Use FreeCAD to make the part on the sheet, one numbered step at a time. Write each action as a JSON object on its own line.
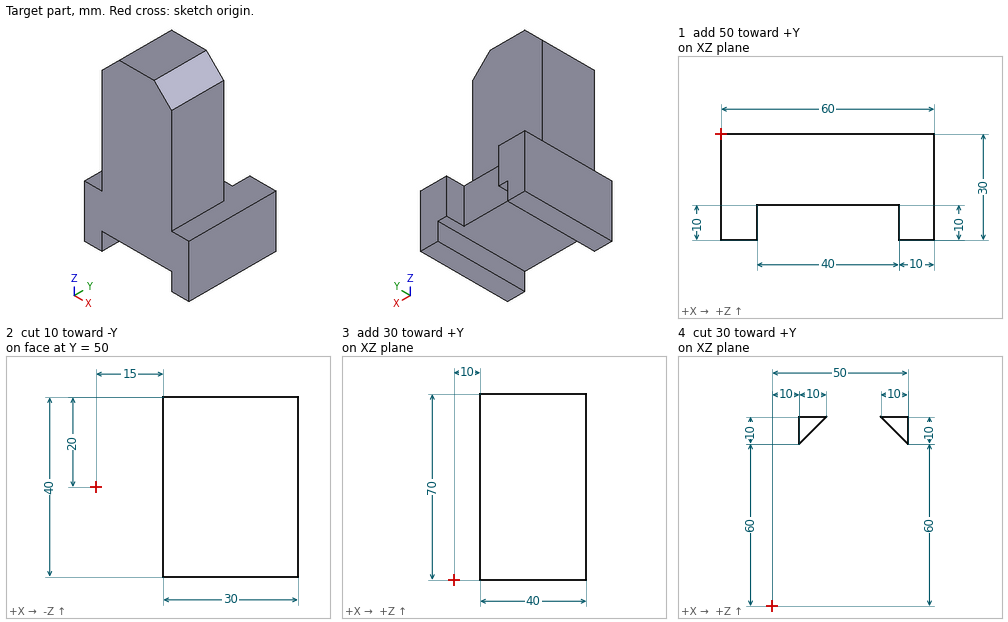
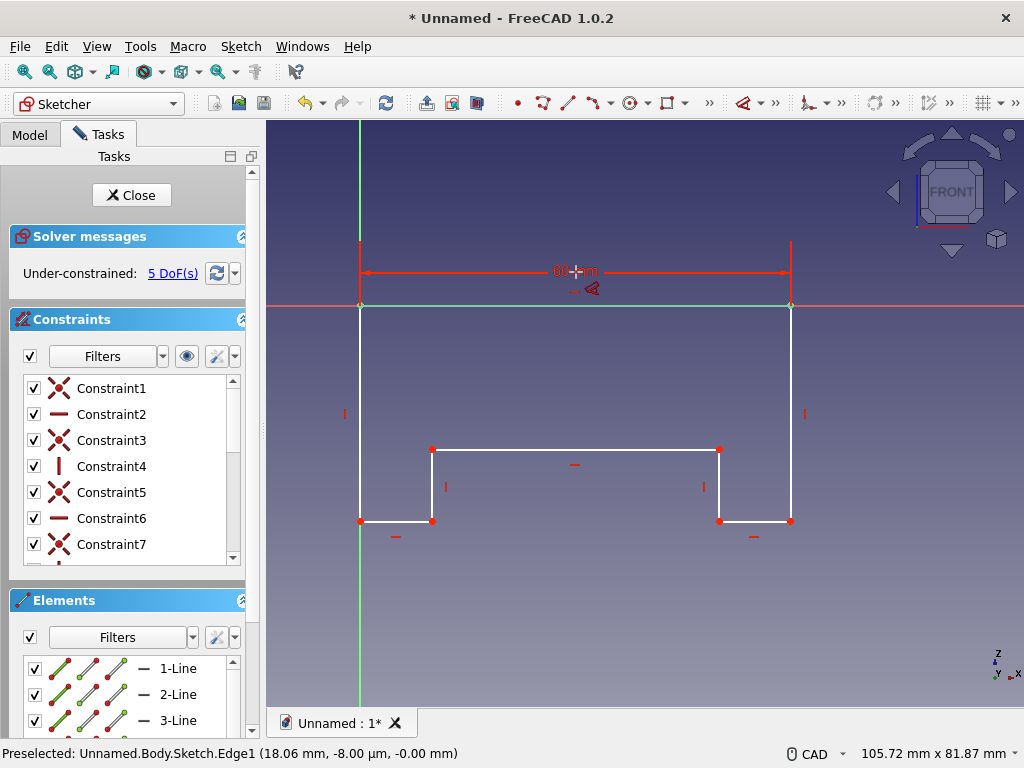
{"action": "left_click", "coordinate": [791, 371]}
{"action": "left_click", "coordinate": [825, 414]}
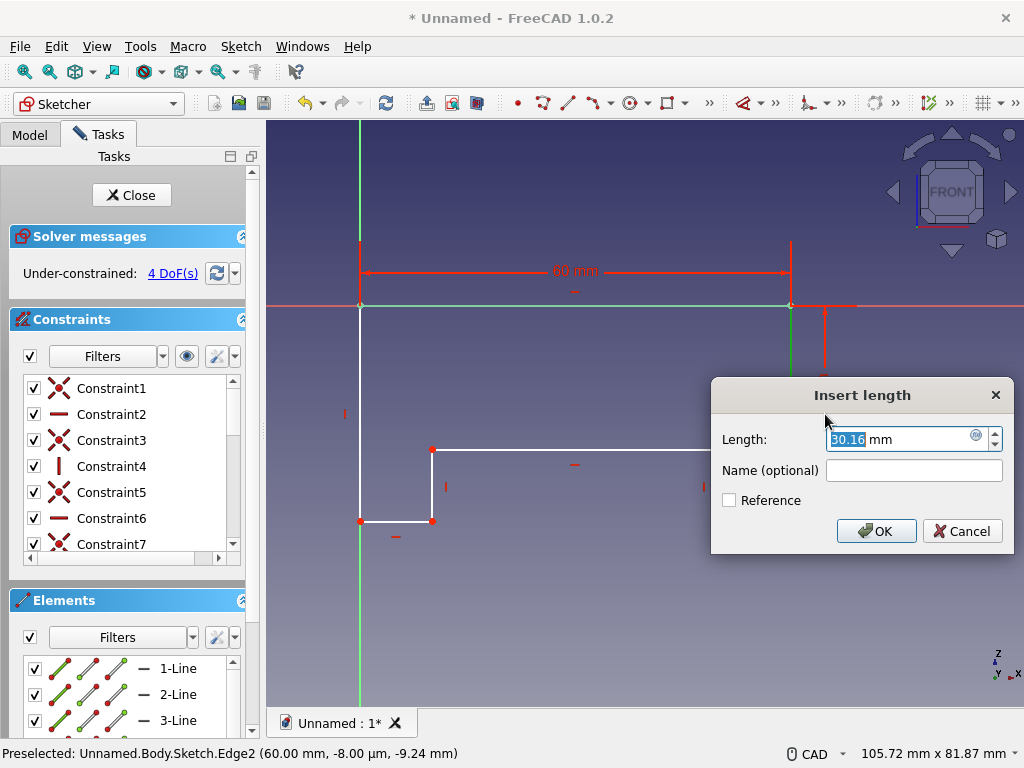
{"action": "type", "text": "30"}
{"action": "key", "text": "Return"}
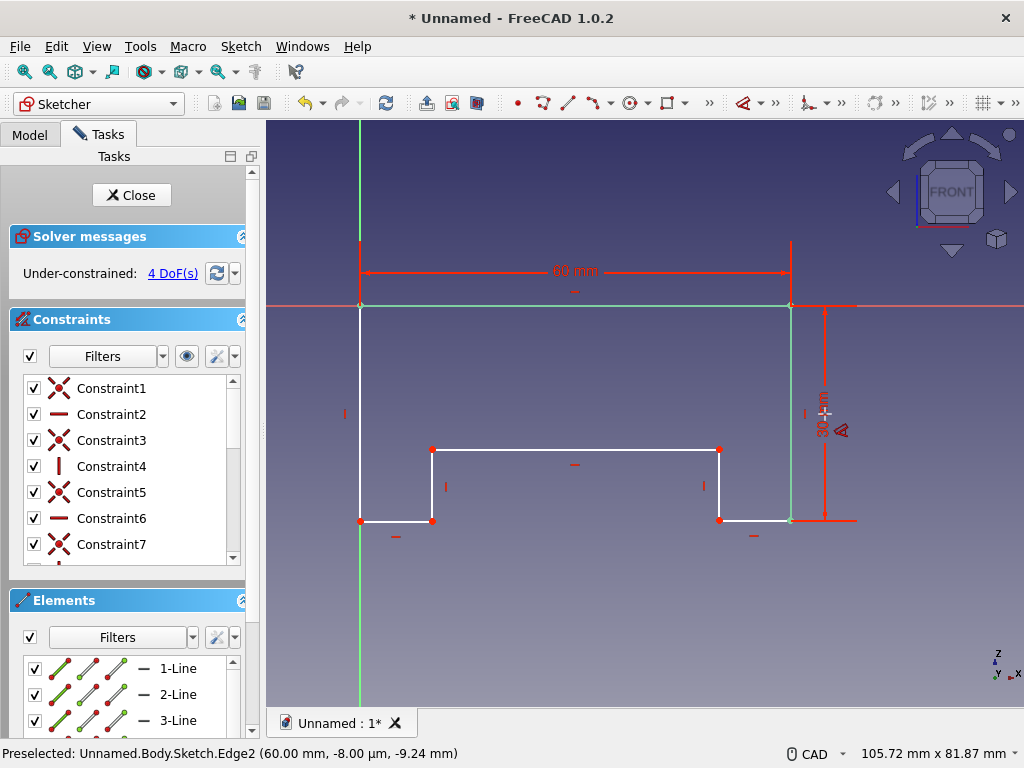
{"action": "left_click", "coordinate": [769, 521]}
{"action": "left_click", "coordinate": [755, 555]}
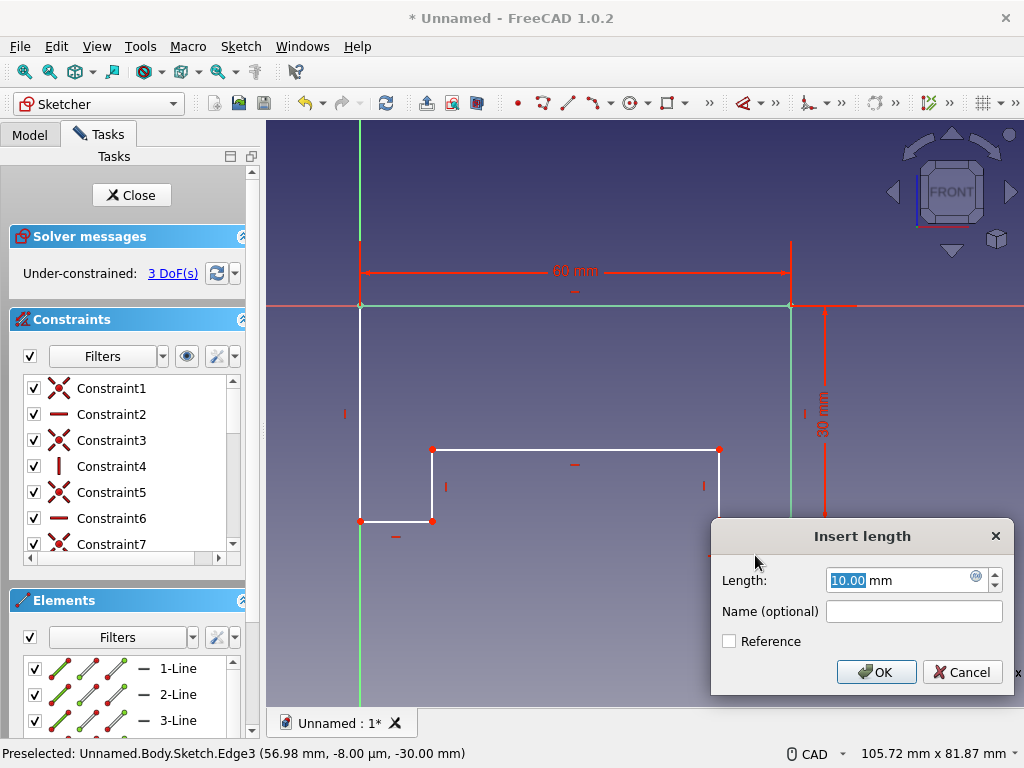
{"action": "type", "text": "10"}
{"action": "key", "text": "Return"}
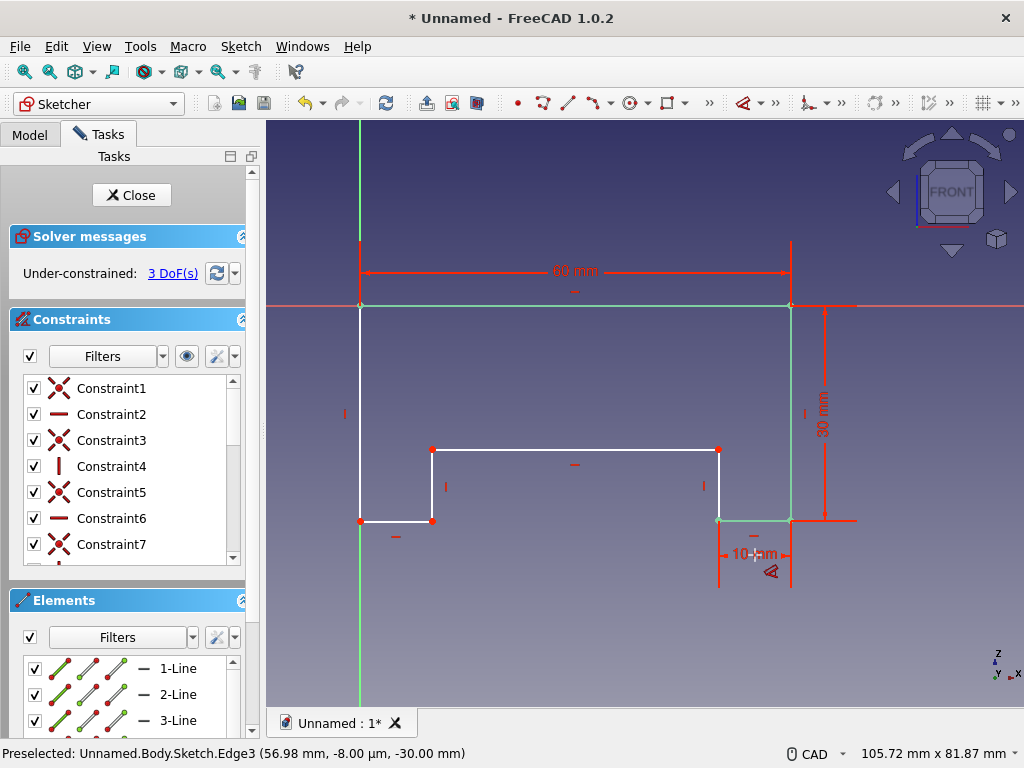
{"action": "left_click", "coordinate": [719, 500]}
{"action": "left_click", "coordinate": [753, 485]}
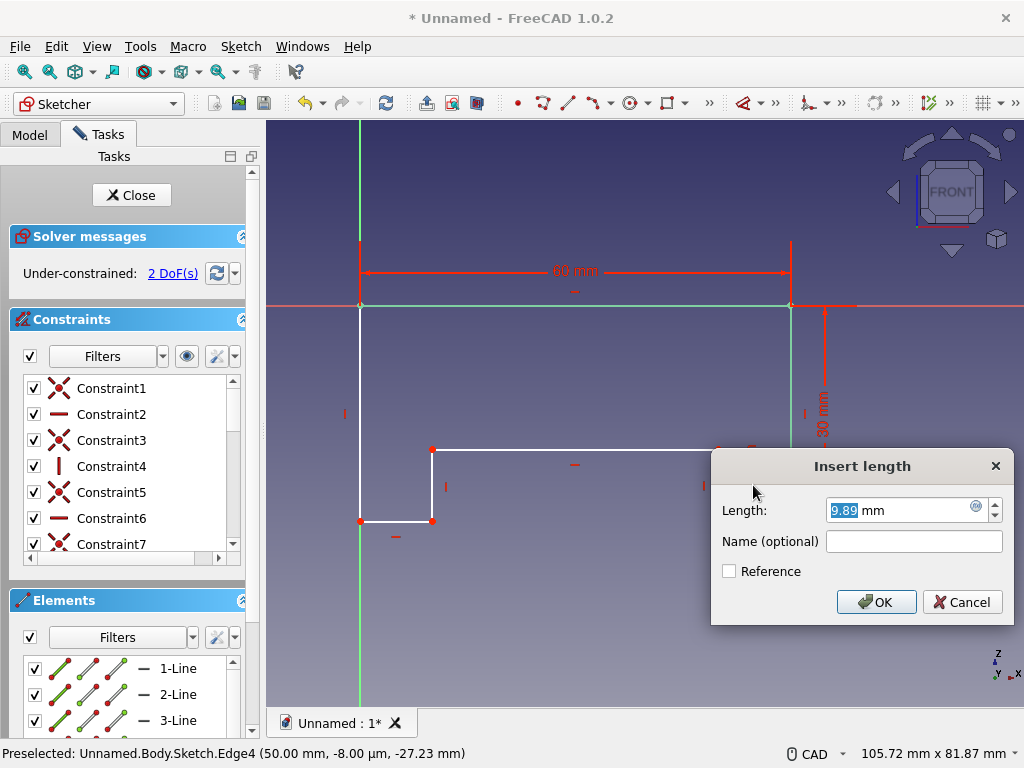
{"action": "type", "text": "10"}
{"action": "key", "text": "Return"}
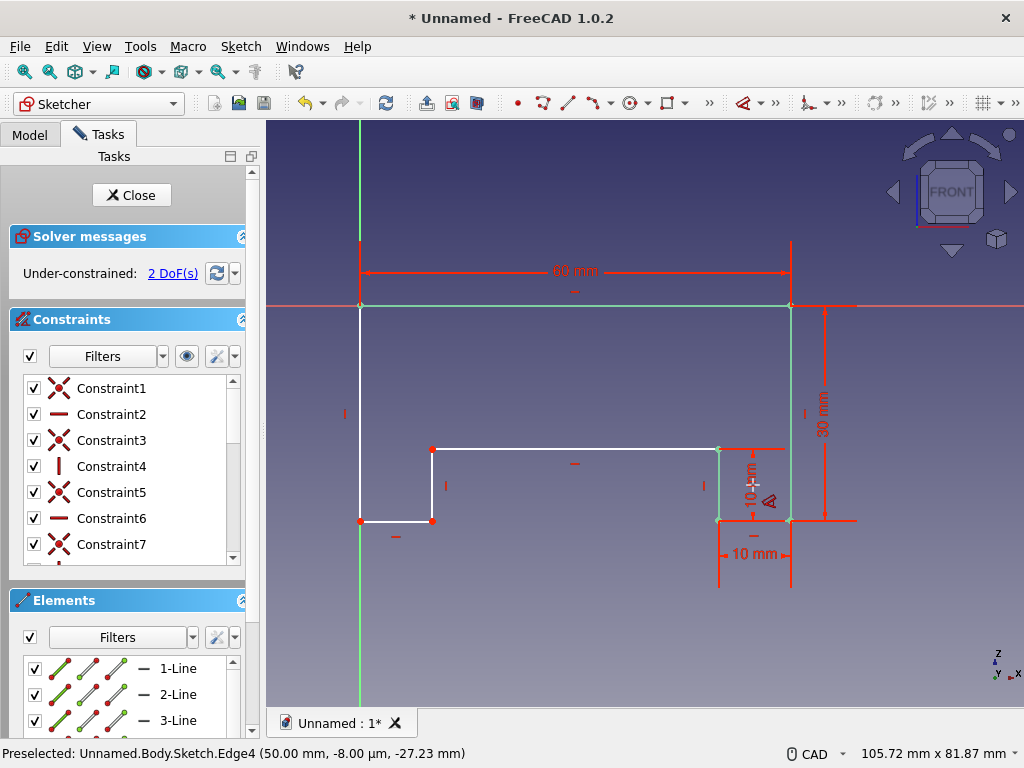
{"action": "left_click", "coordinate": [633, 449]}
{"action": "left_click", "coordinate": [575, 483]}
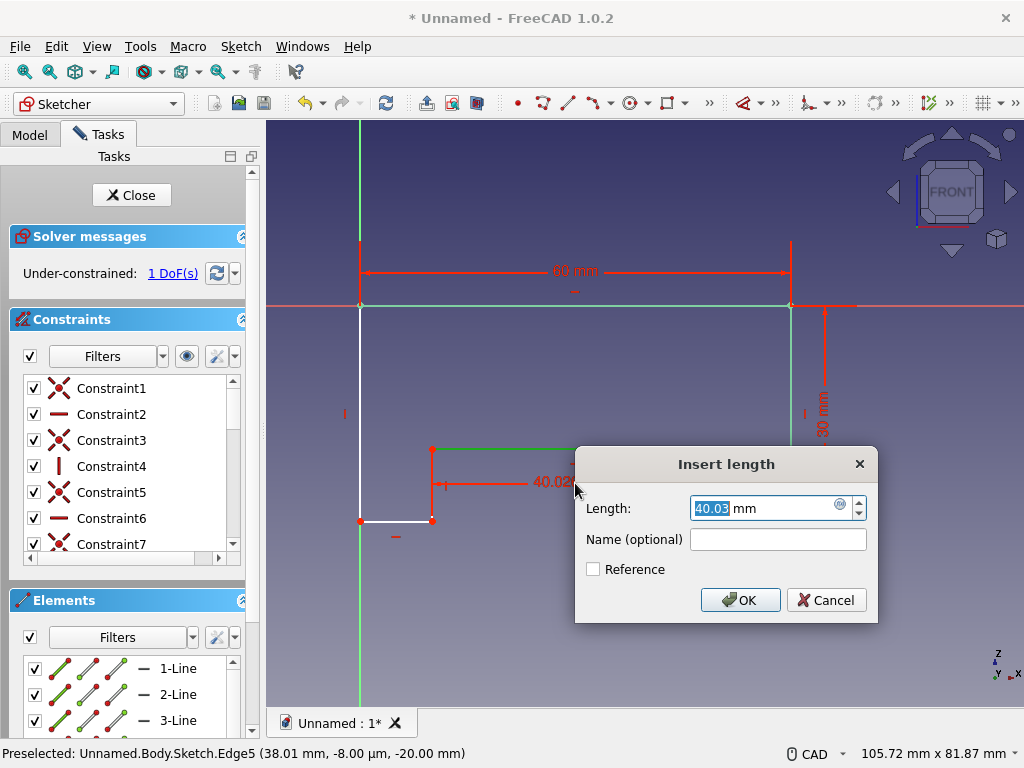
{"action": "type", "text": "40"}
{"action": "key", "text": "Return"}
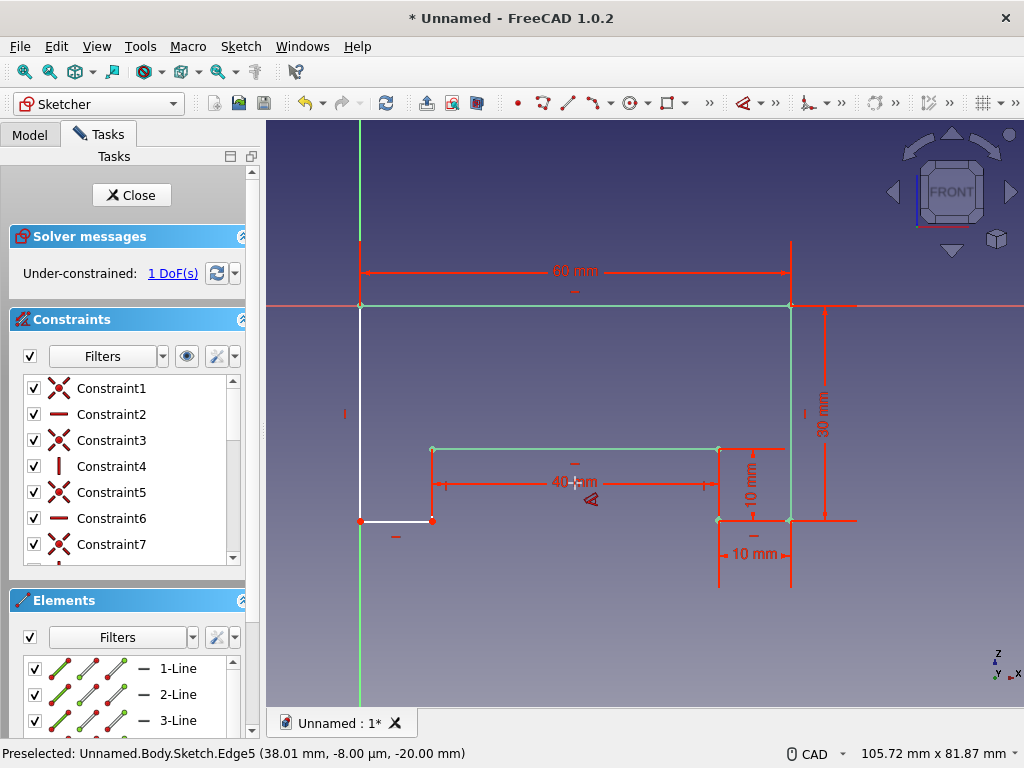
{"action": "left_click", "coordinate": [432, 471]}
{"action": "left_click", "coordinate": [398, 486]}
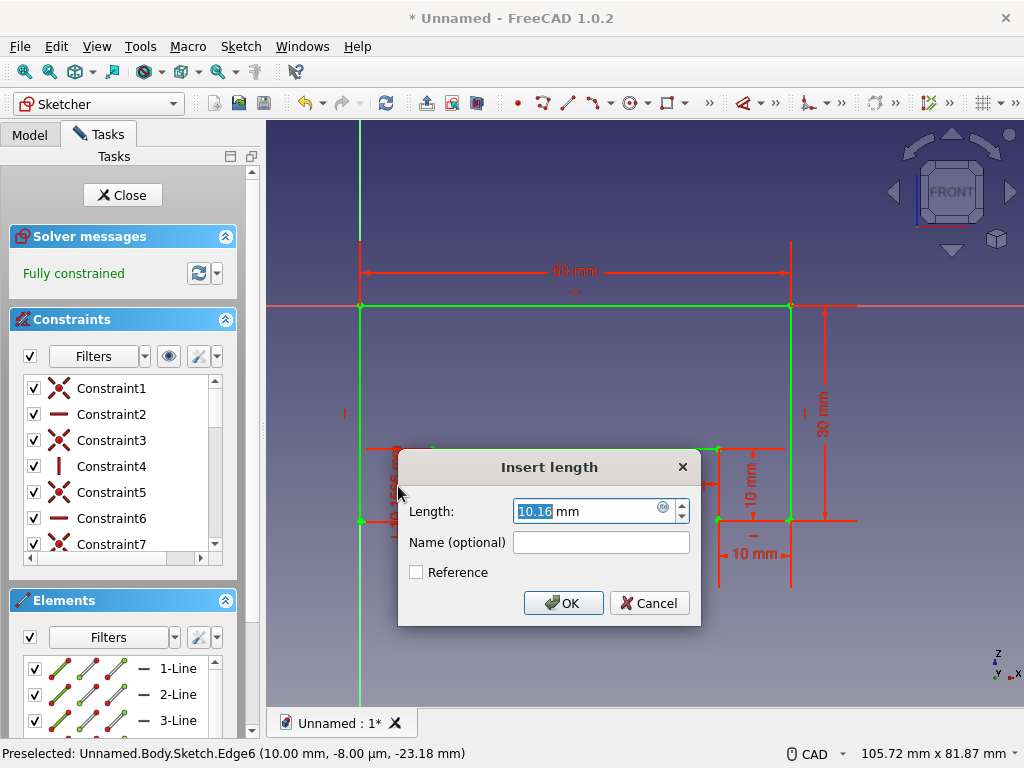
{"action": "type", "text": "10"}
{"action": "key", "text": "Return"}
{"action": "key", "text": "Escape"}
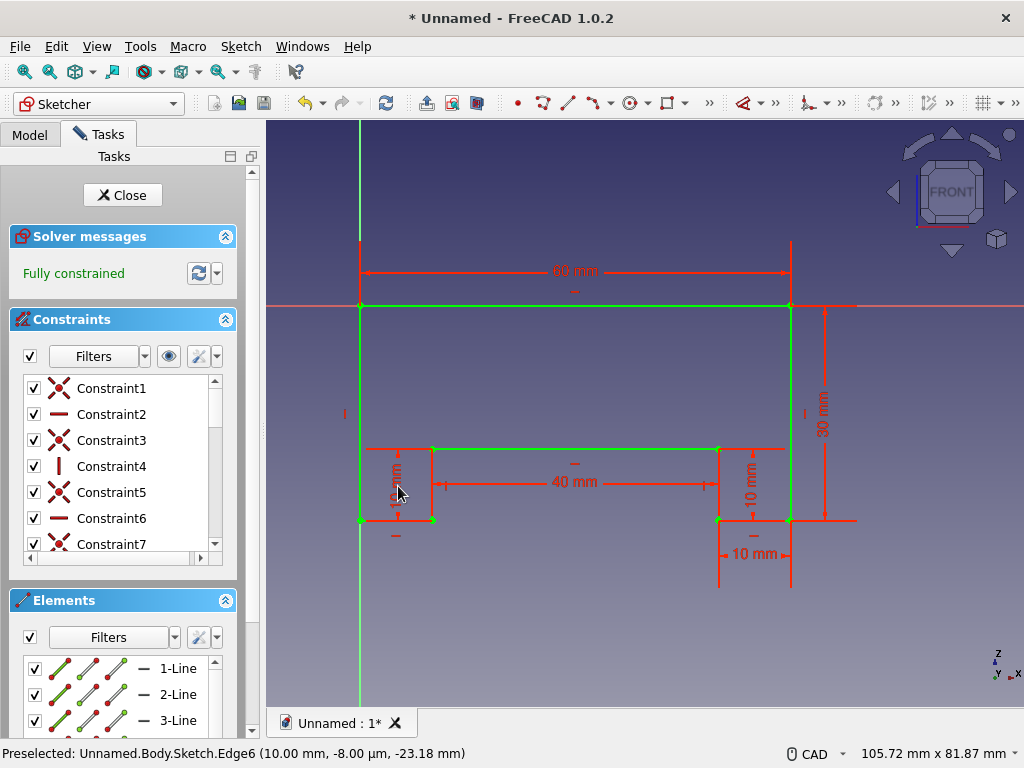
{"action": "left_click", "coordinate": [123, 195]}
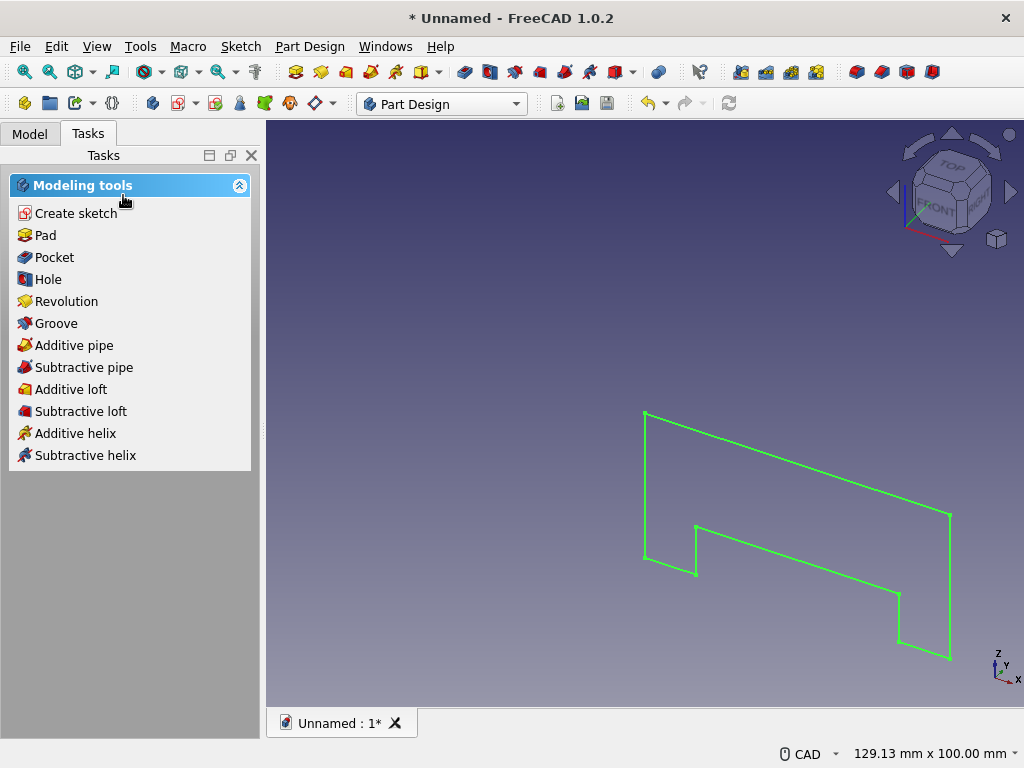
{"action": "left_click", "coordinate": [296, 72]}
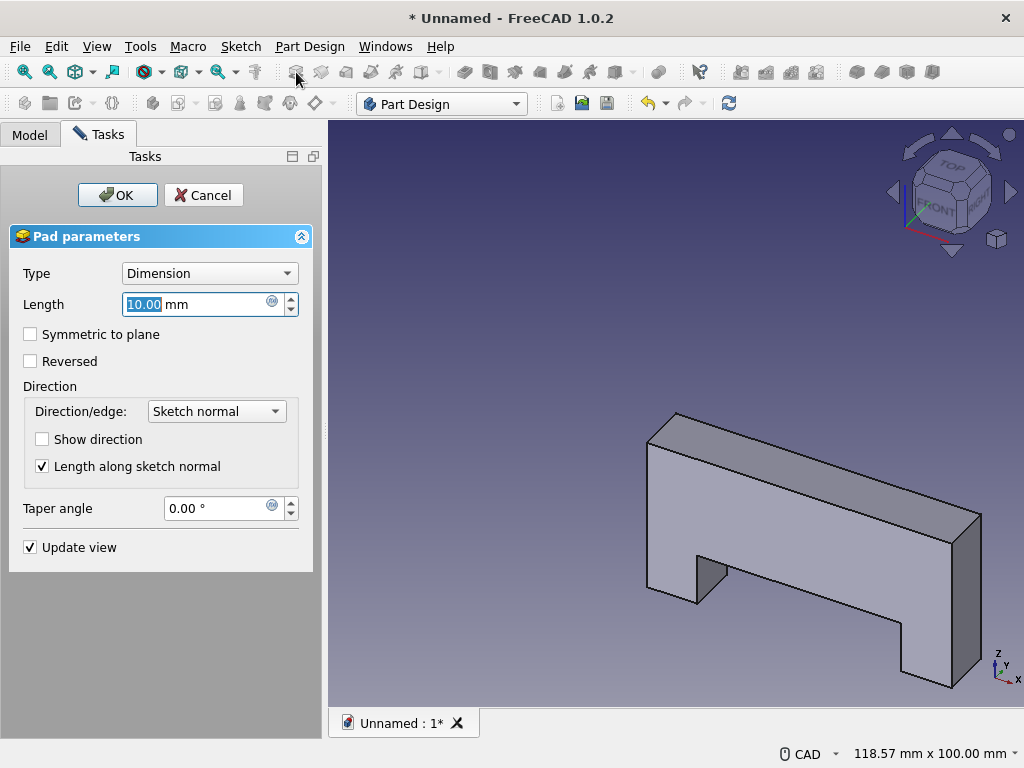
{"action": "type", "text": "50"}
{"action": "key", "text": "Tab"}